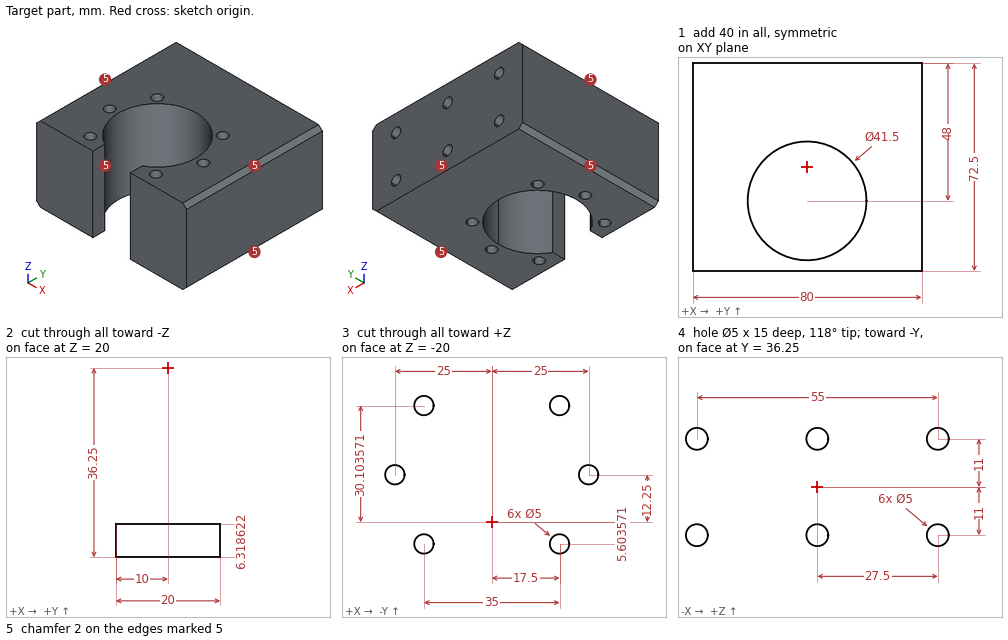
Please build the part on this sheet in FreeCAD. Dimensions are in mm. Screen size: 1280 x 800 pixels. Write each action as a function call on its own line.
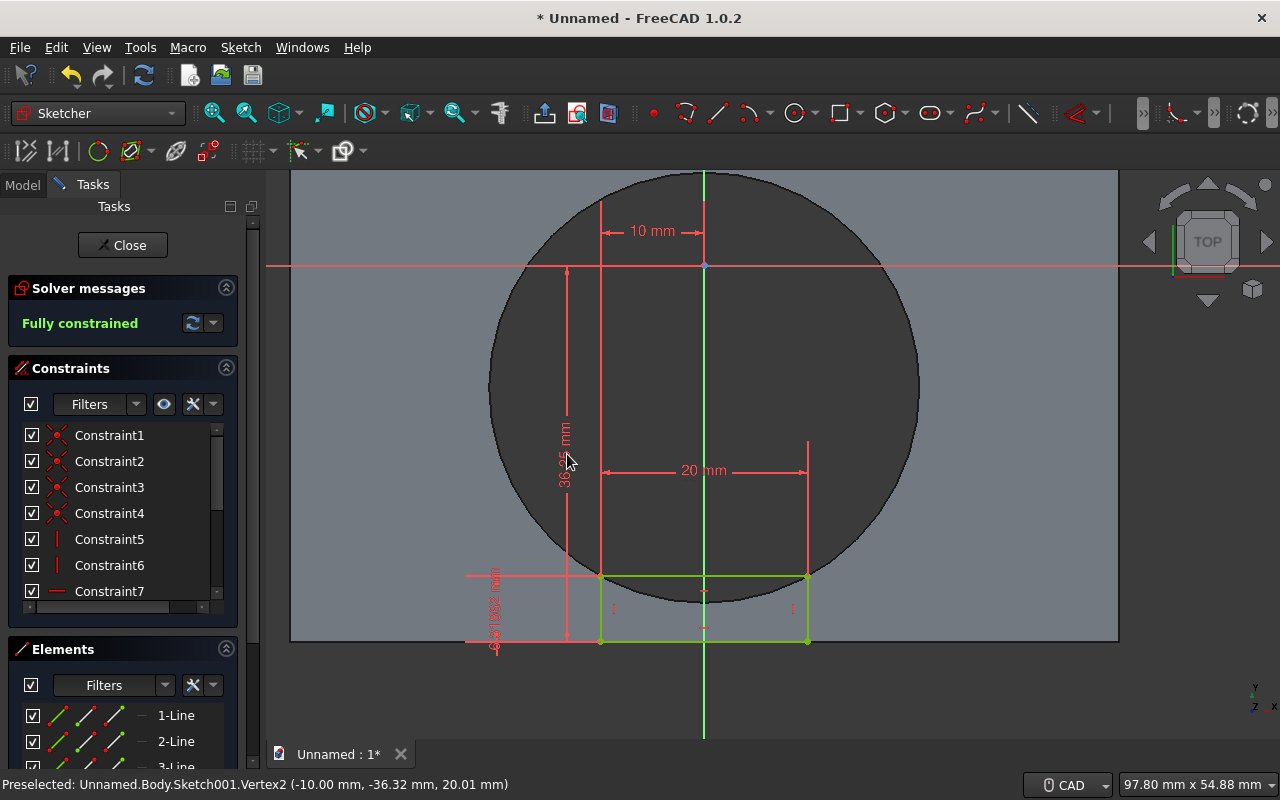
click(123, 245)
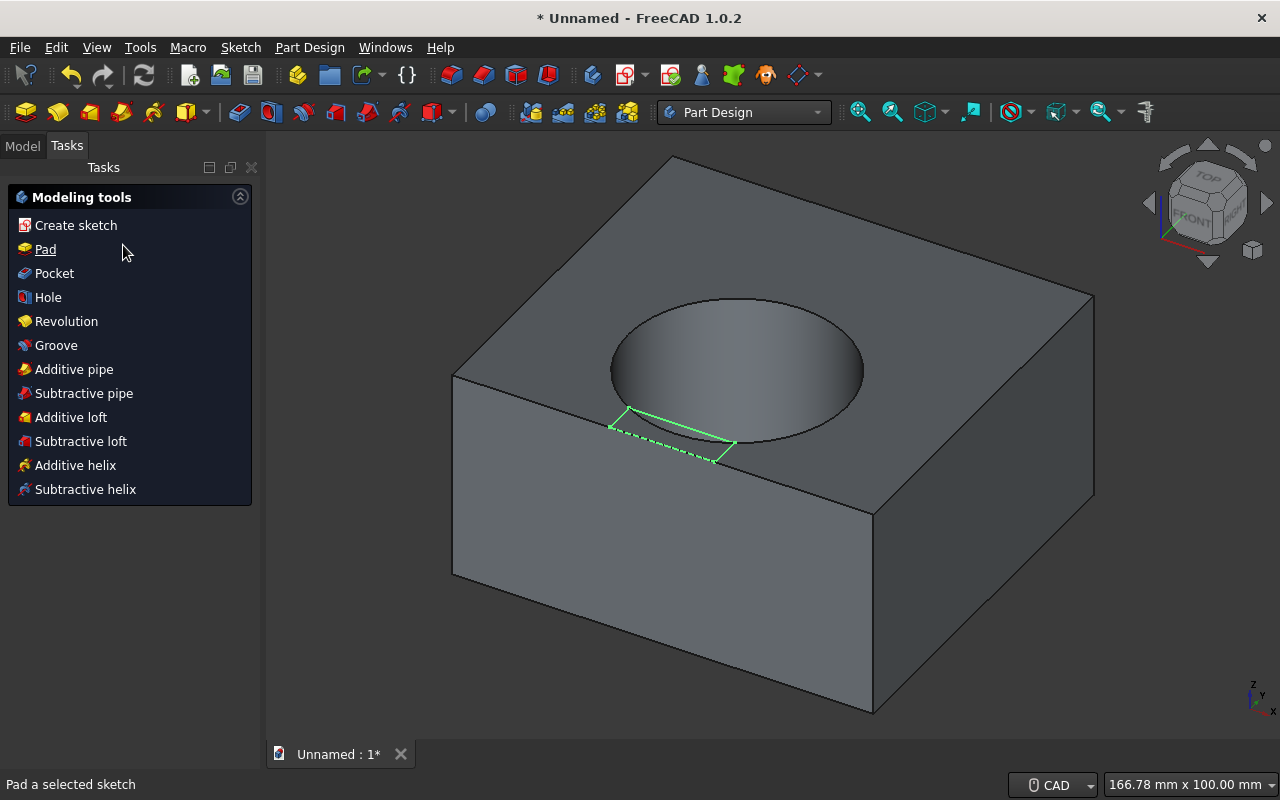
click(240, 112)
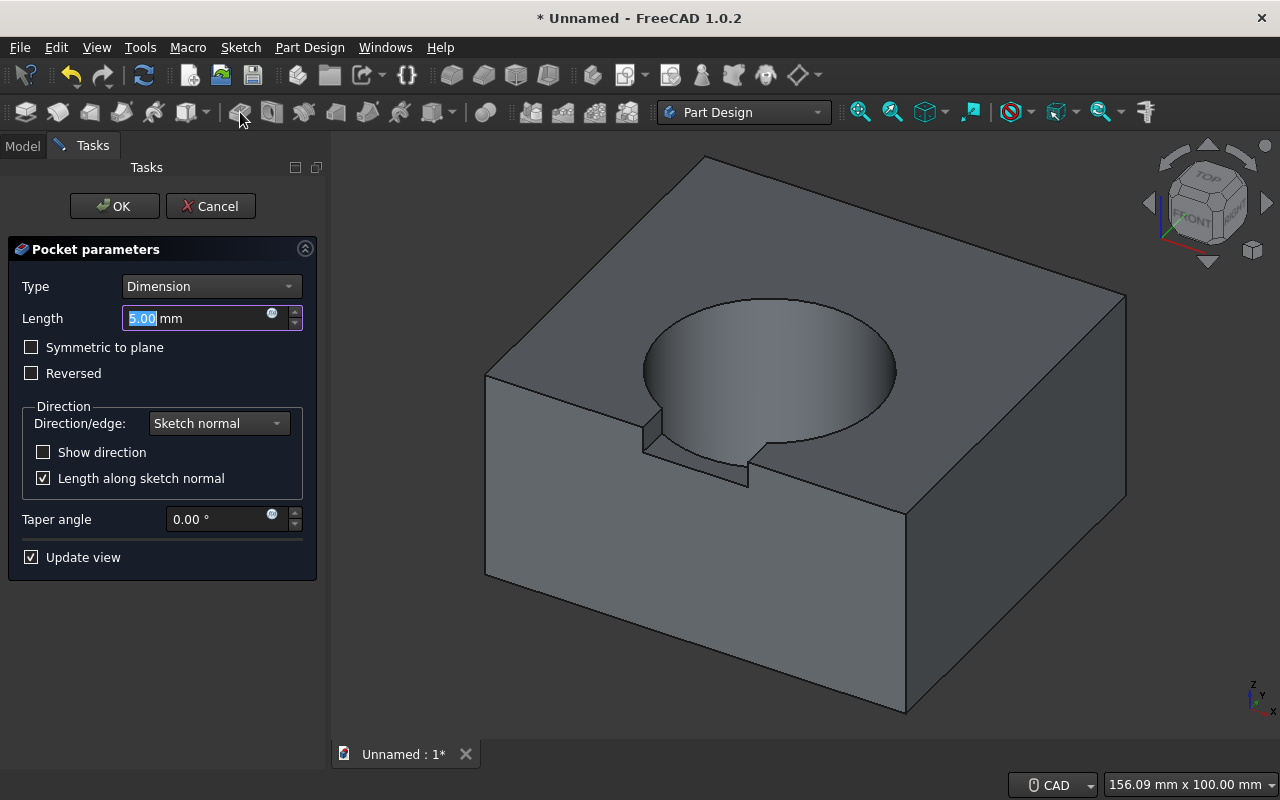
click(212, 286)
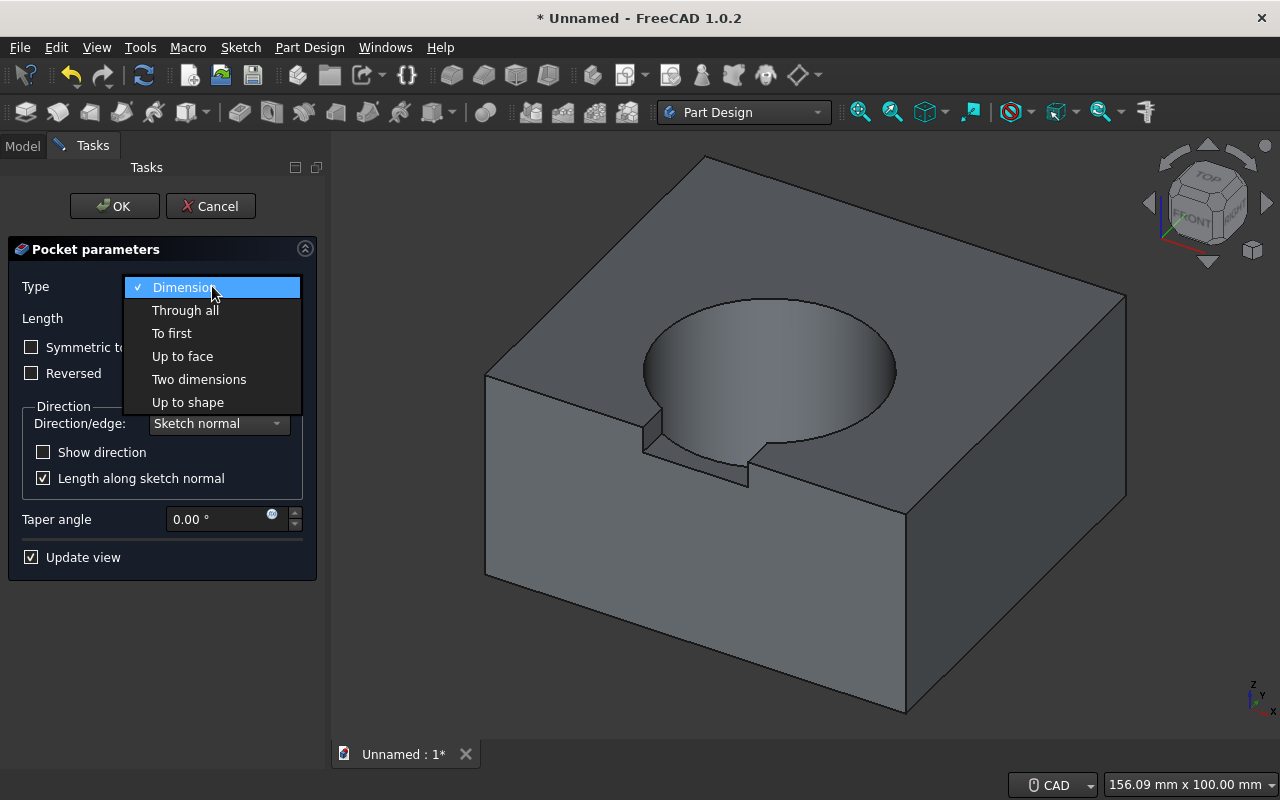
click(212, 310)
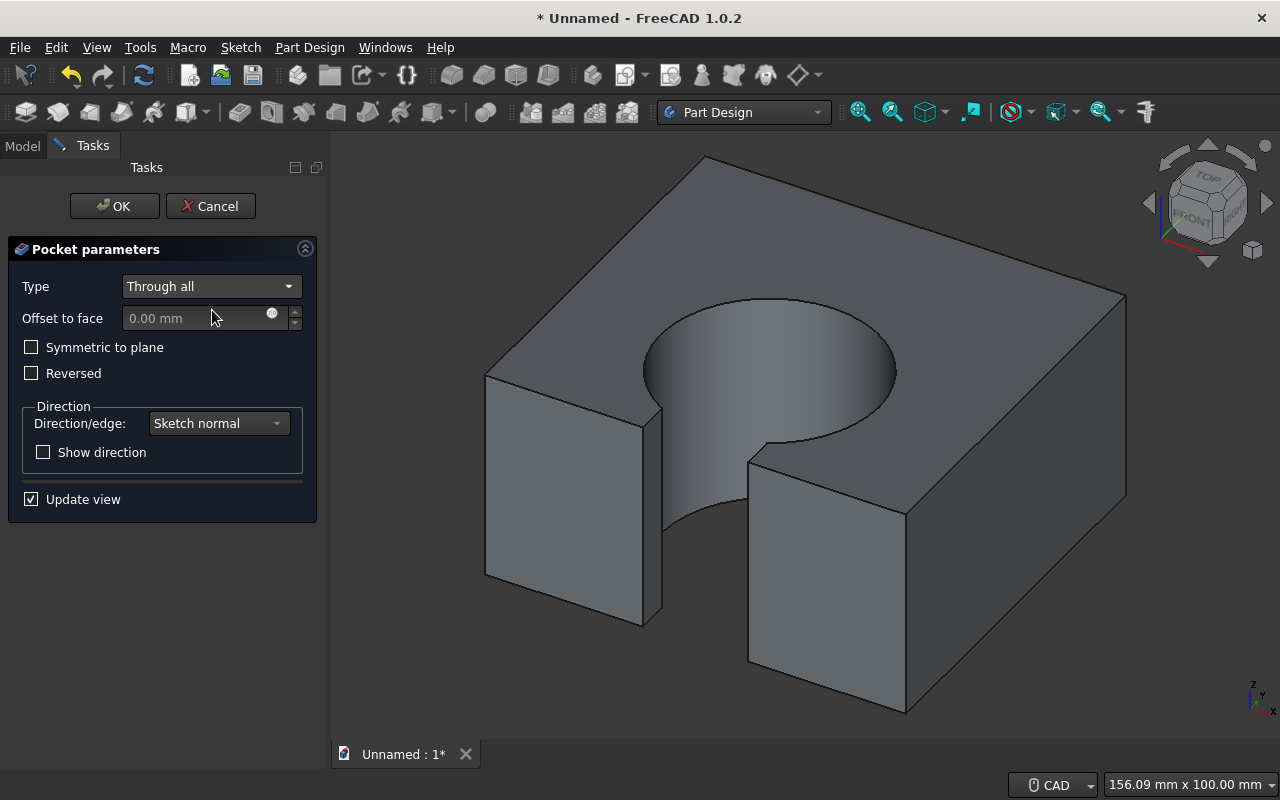
click(115, 206)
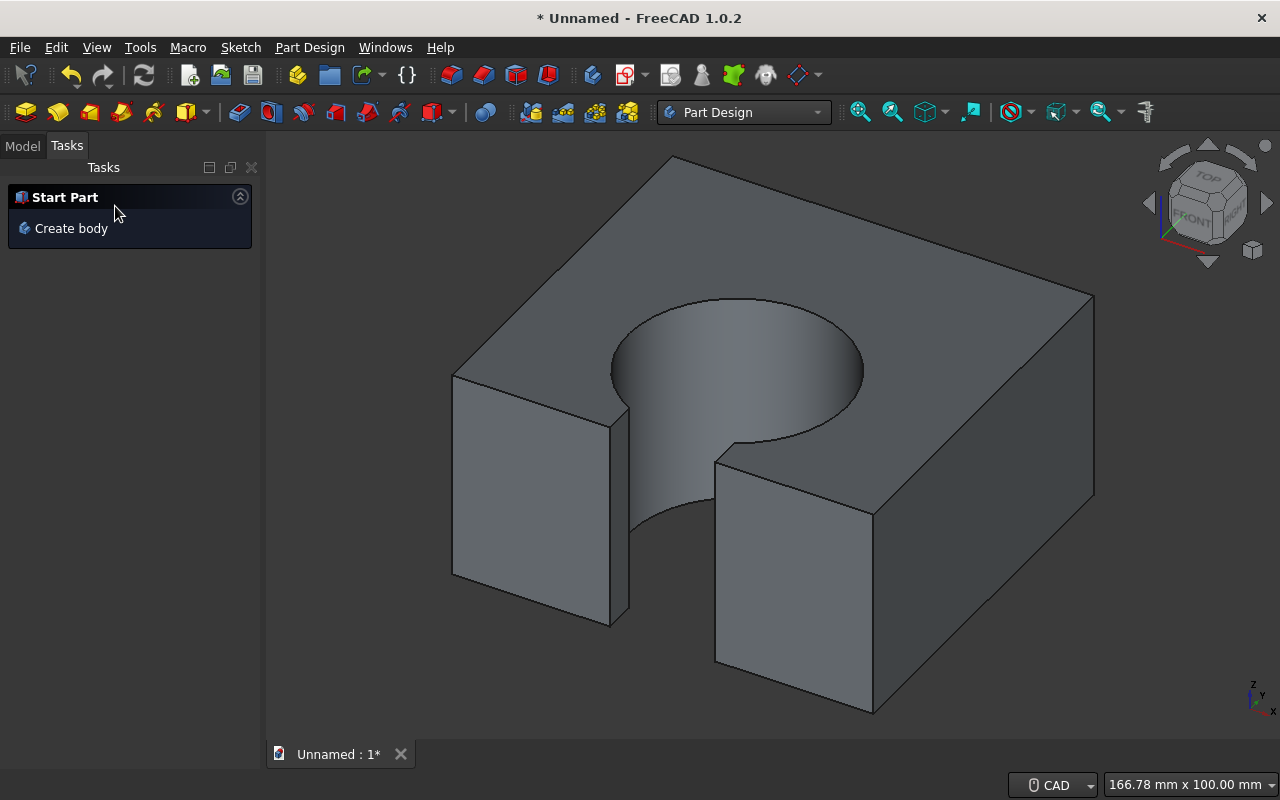
key(5)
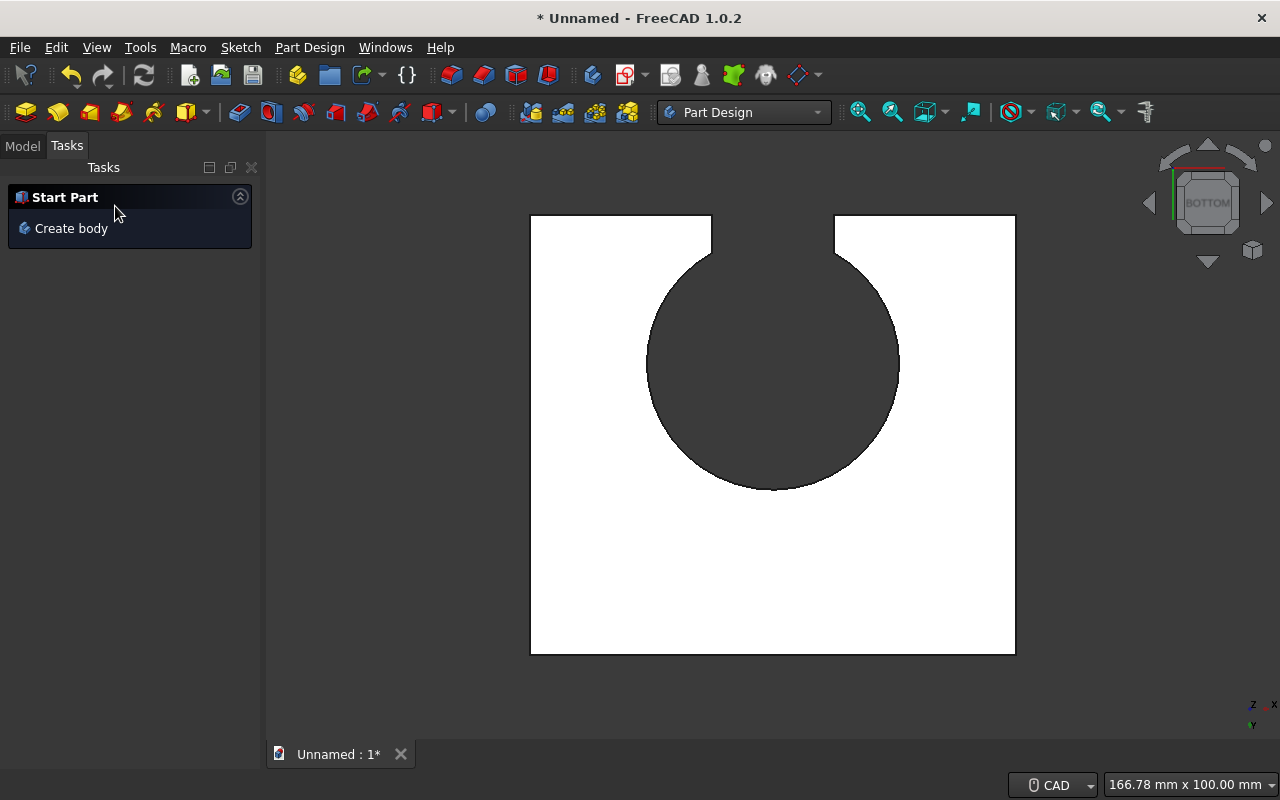
click(912, 560)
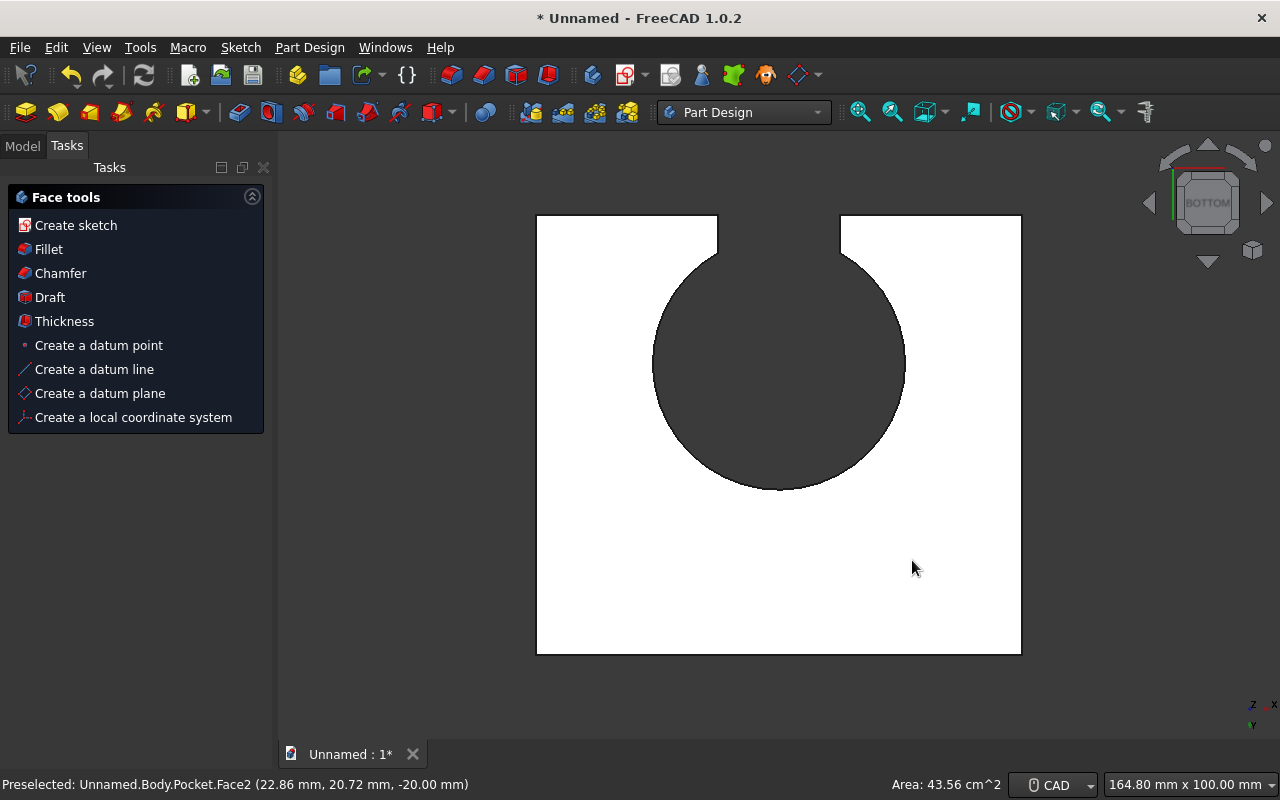
click(626, 76)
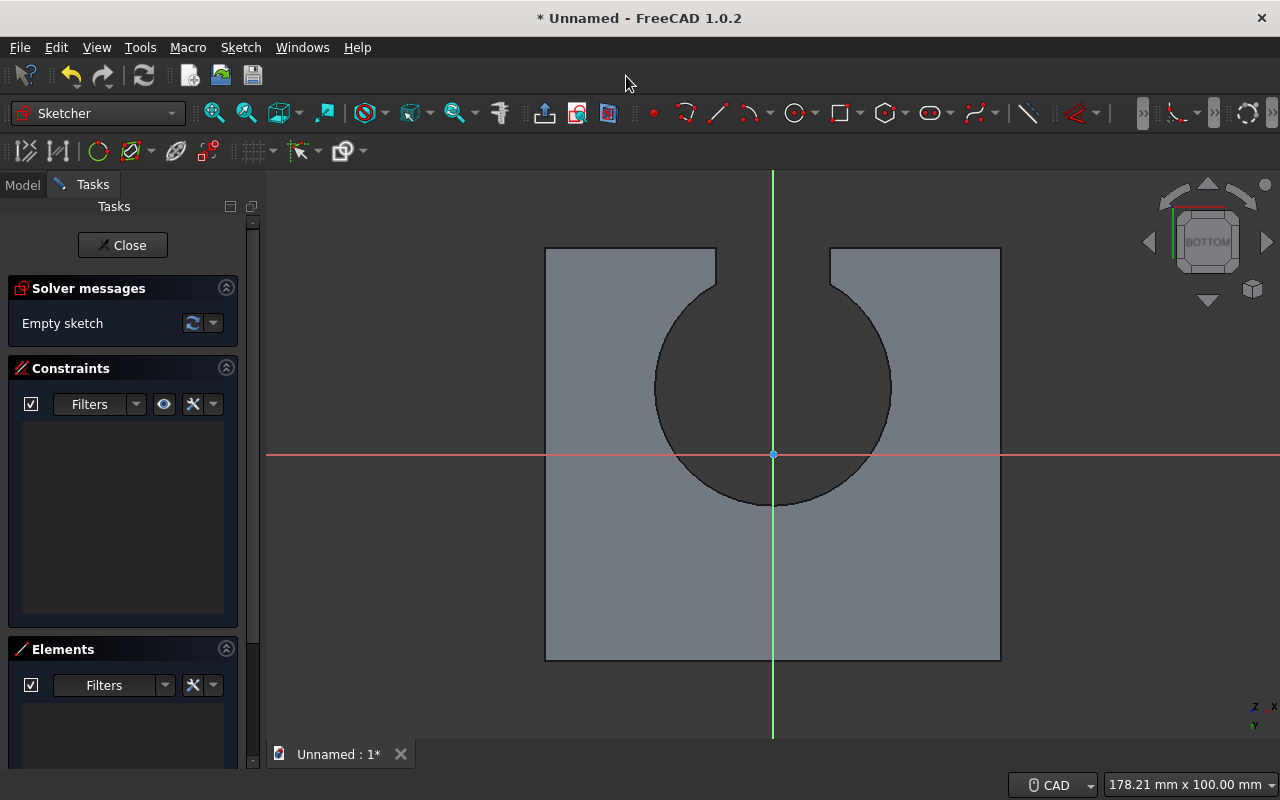
scroll(912, 243, up, 2)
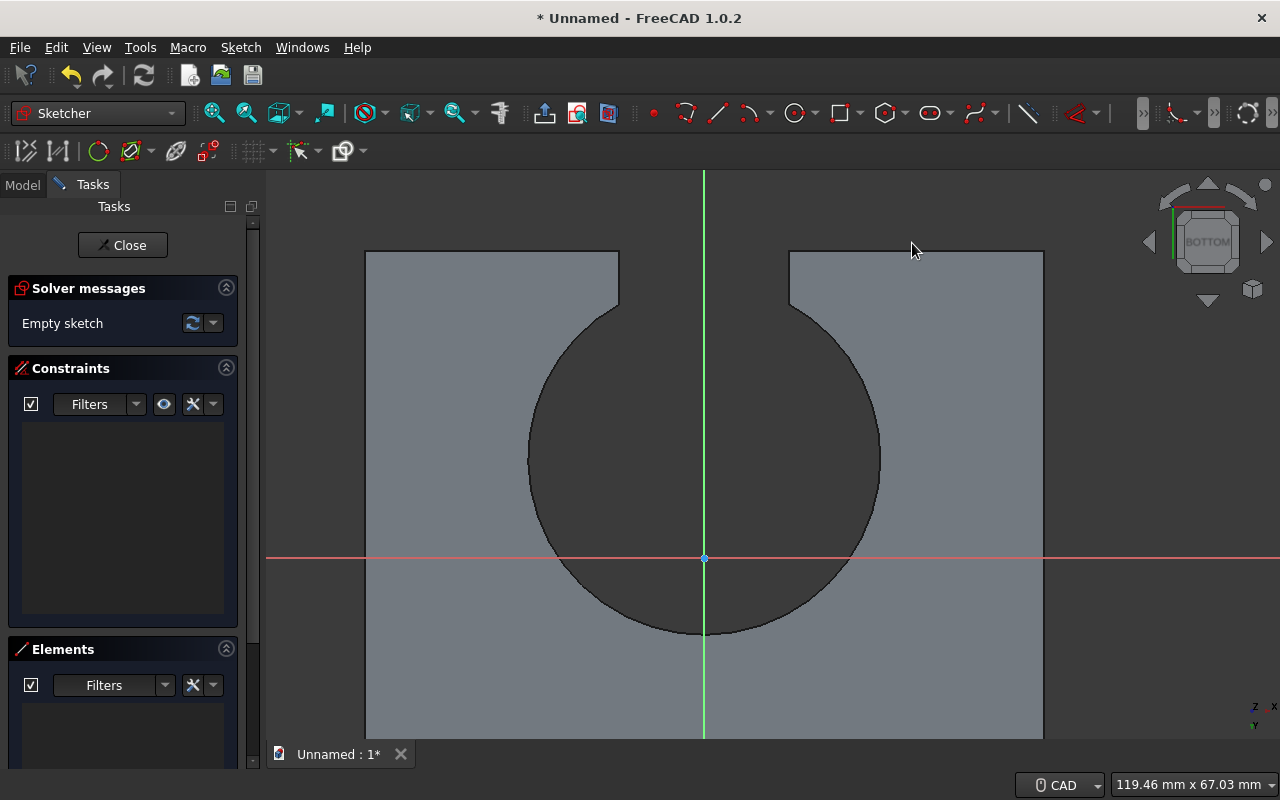
click(796, 114)